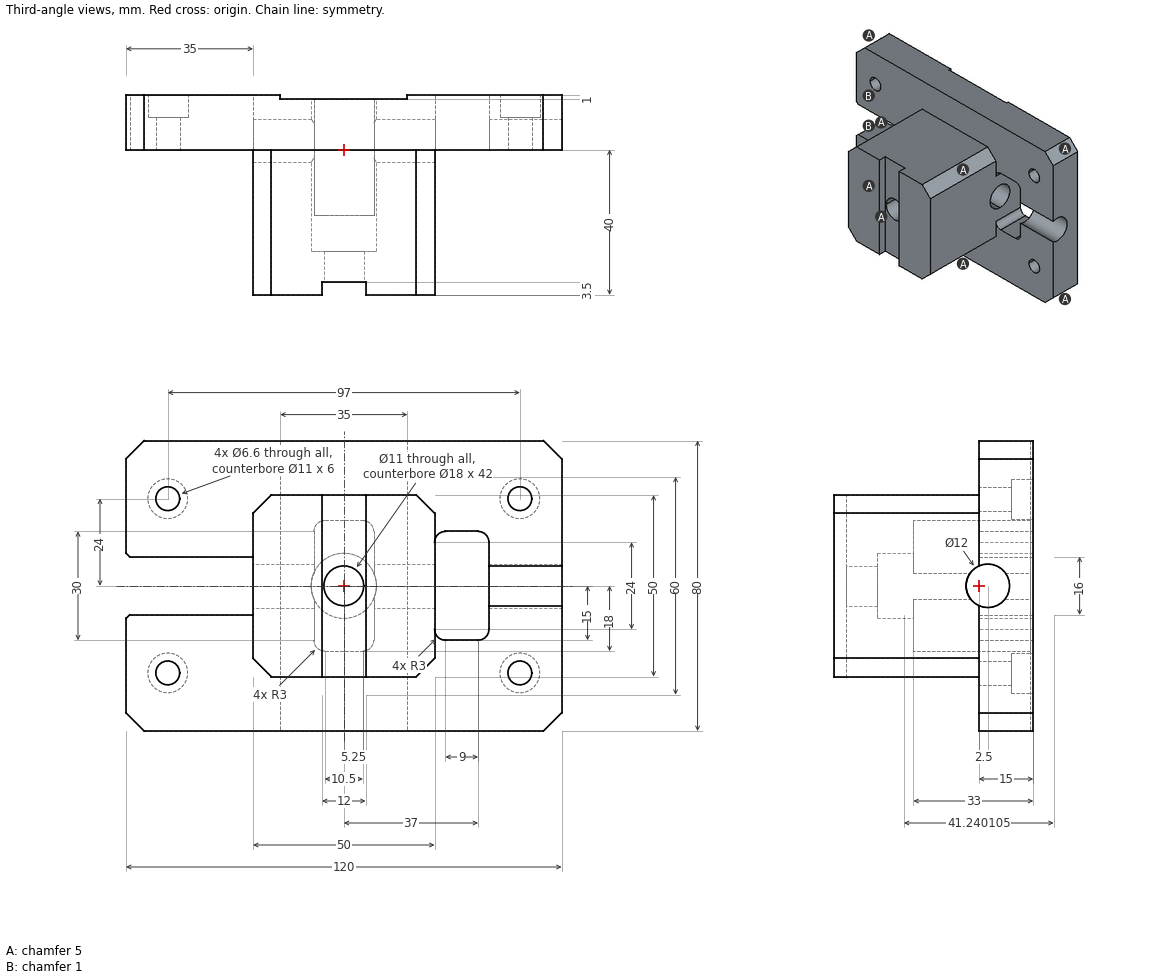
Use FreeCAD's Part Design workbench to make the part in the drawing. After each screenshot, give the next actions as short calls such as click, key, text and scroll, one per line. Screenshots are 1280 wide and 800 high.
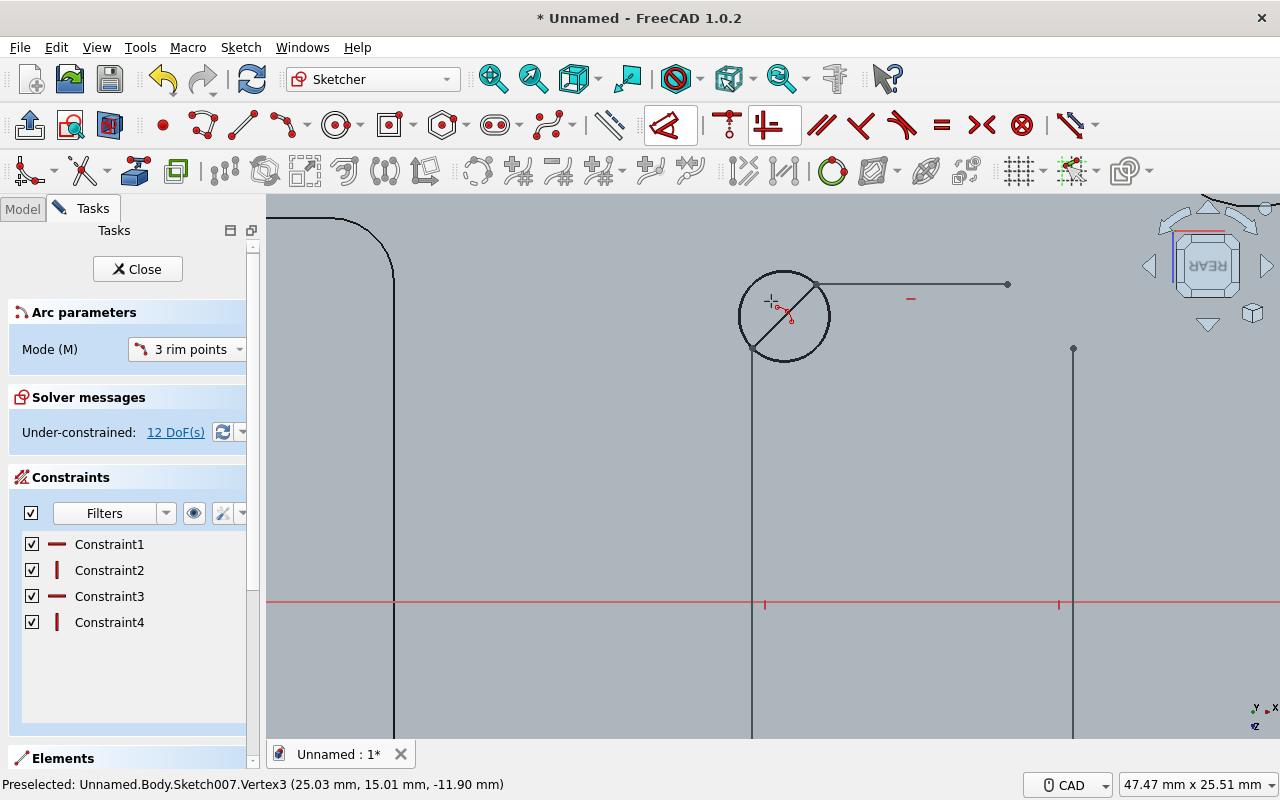
click(771, 301)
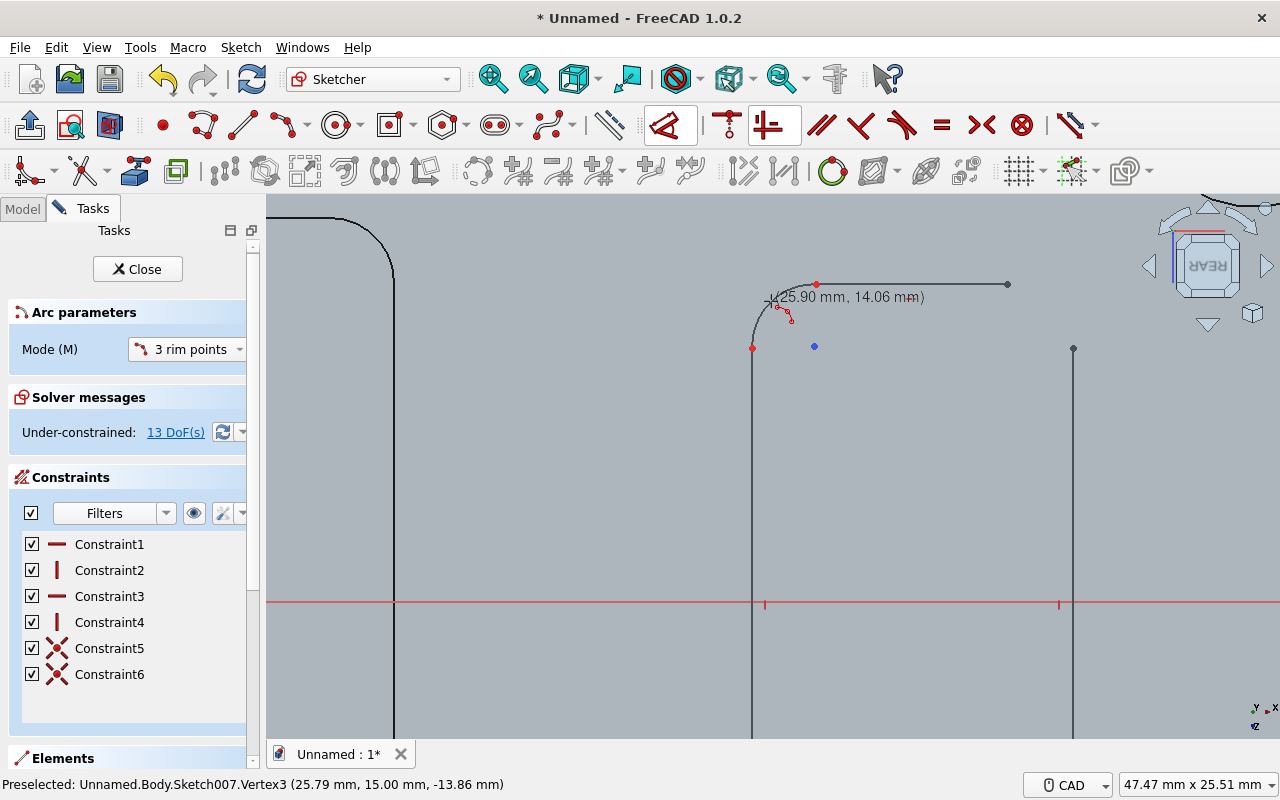
scroll(777, 301, down, 3)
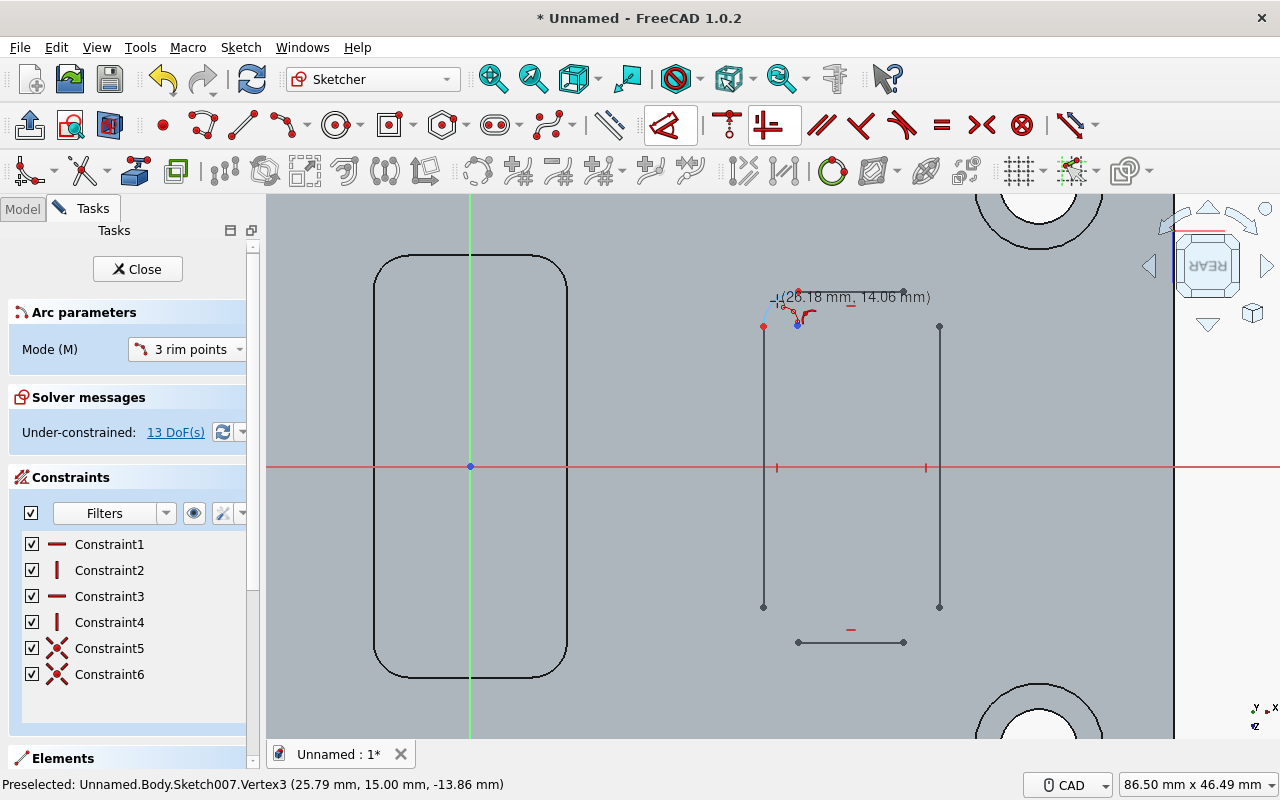
click(764, 608)
click(799, 643)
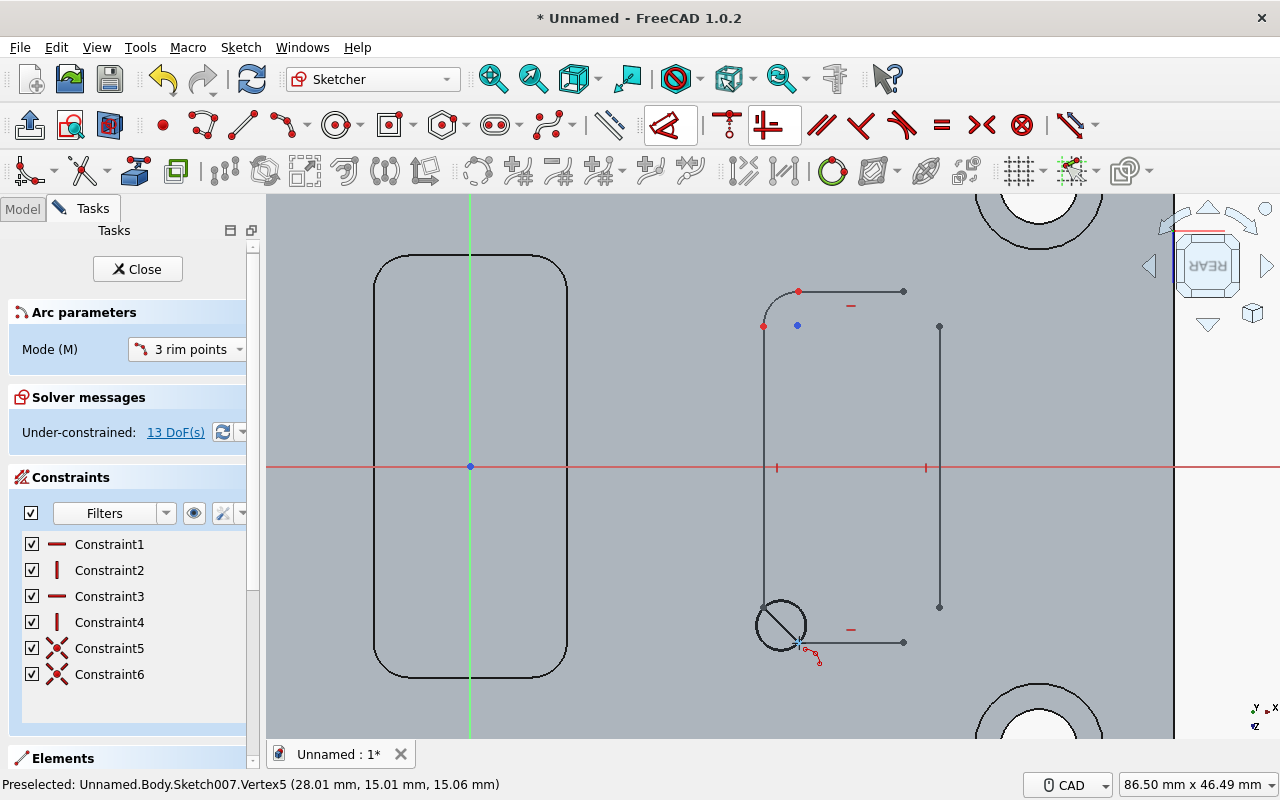
scroll(774, 632, up, 3)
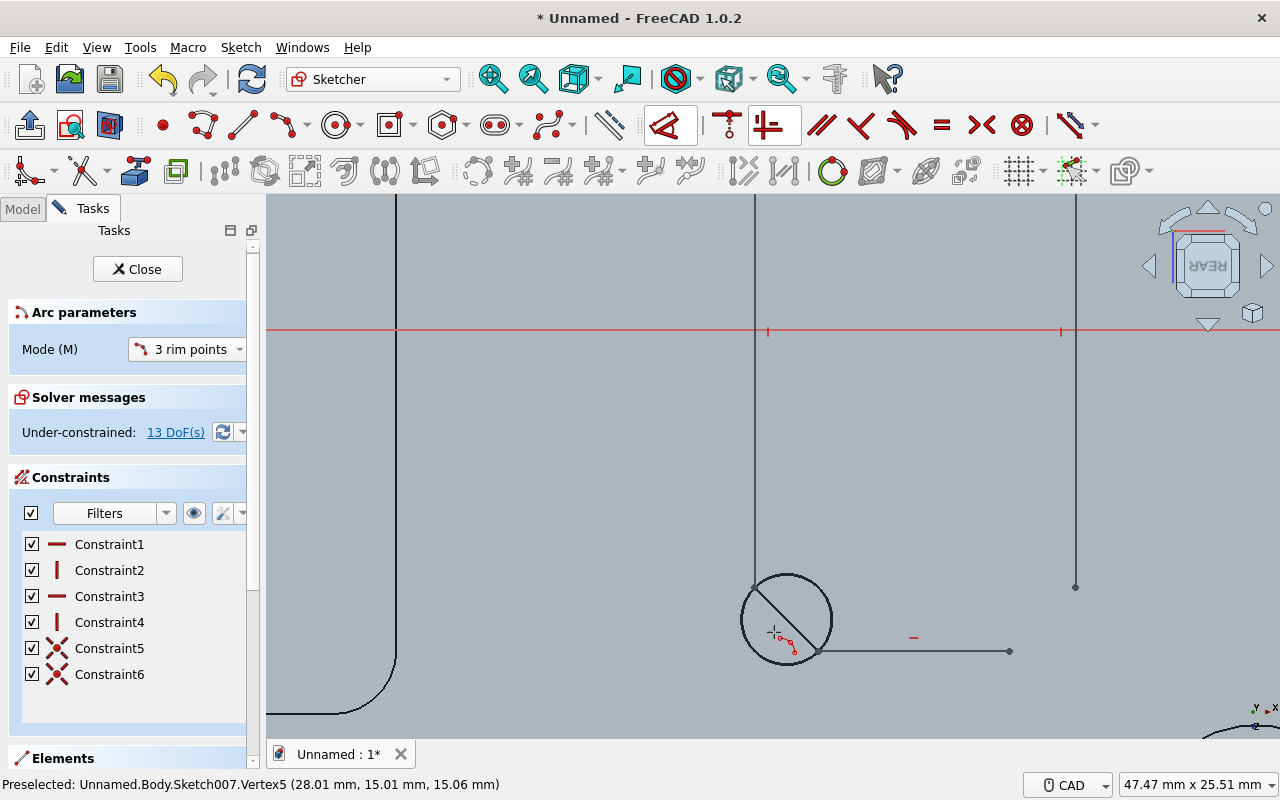
click(773, 631)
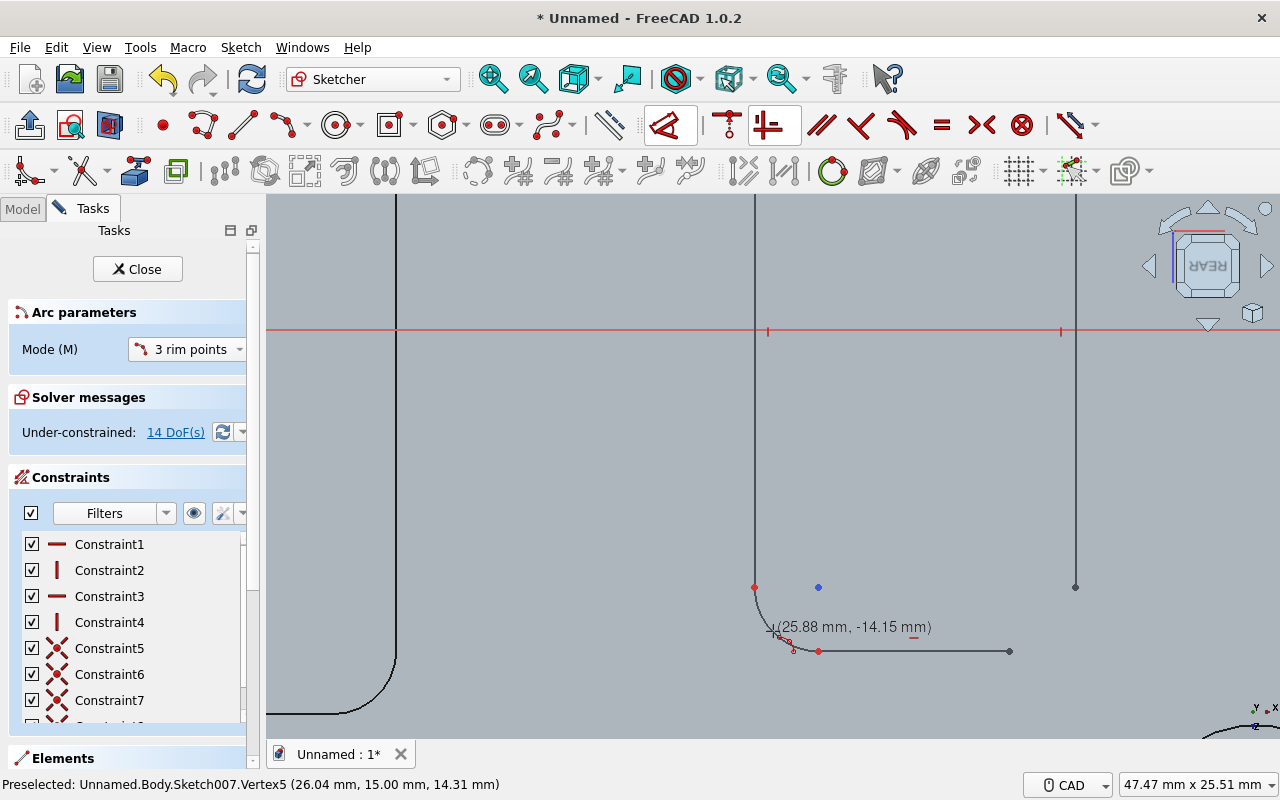
click(1010, 651)
click(1076, 588)
click(1056, 631)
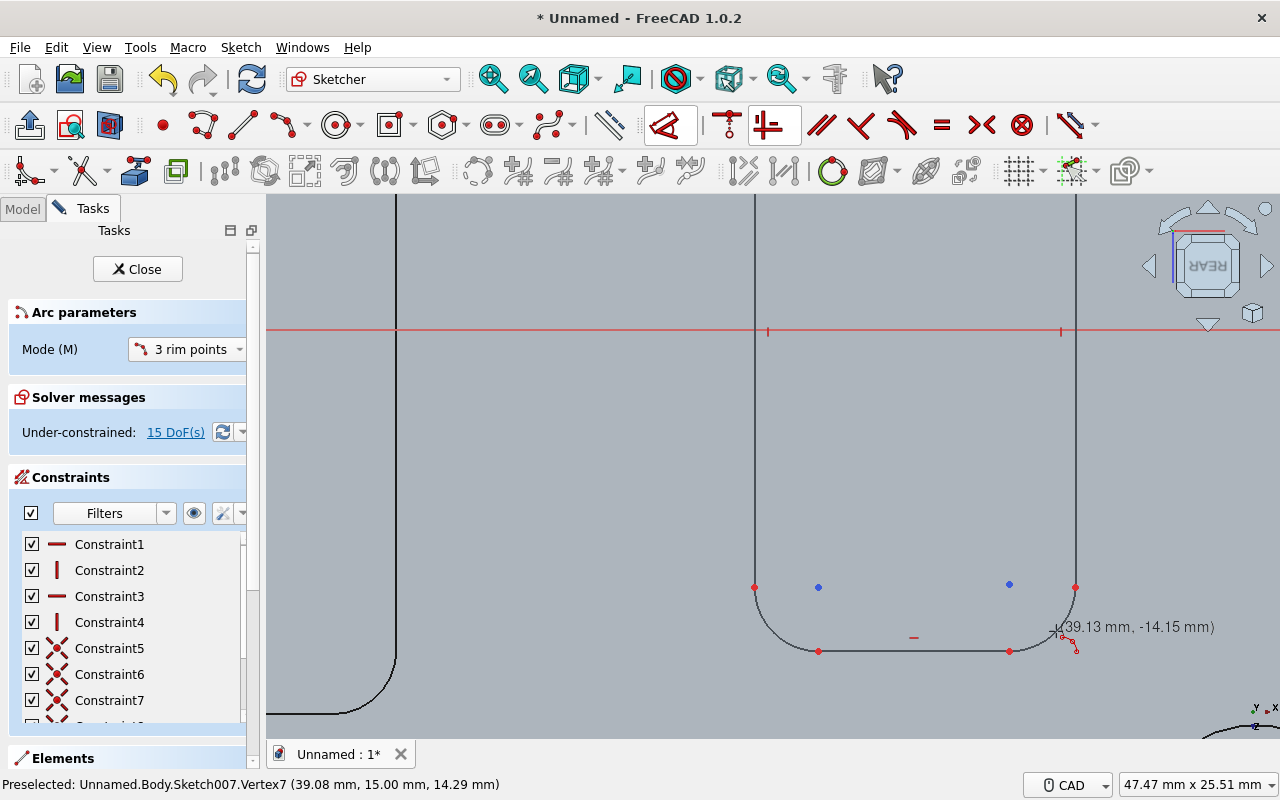
scroll(774, 633, down, 3)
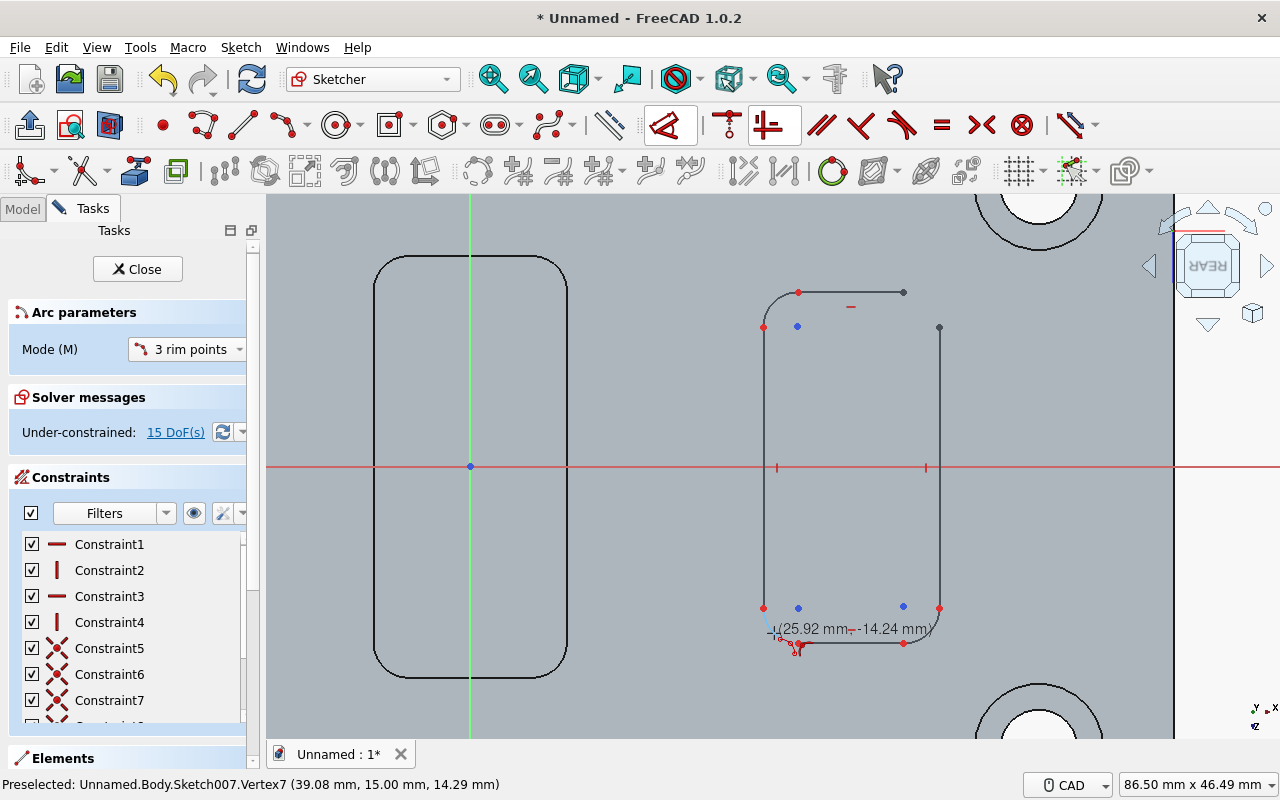
click(940, 327)
click(904, 292)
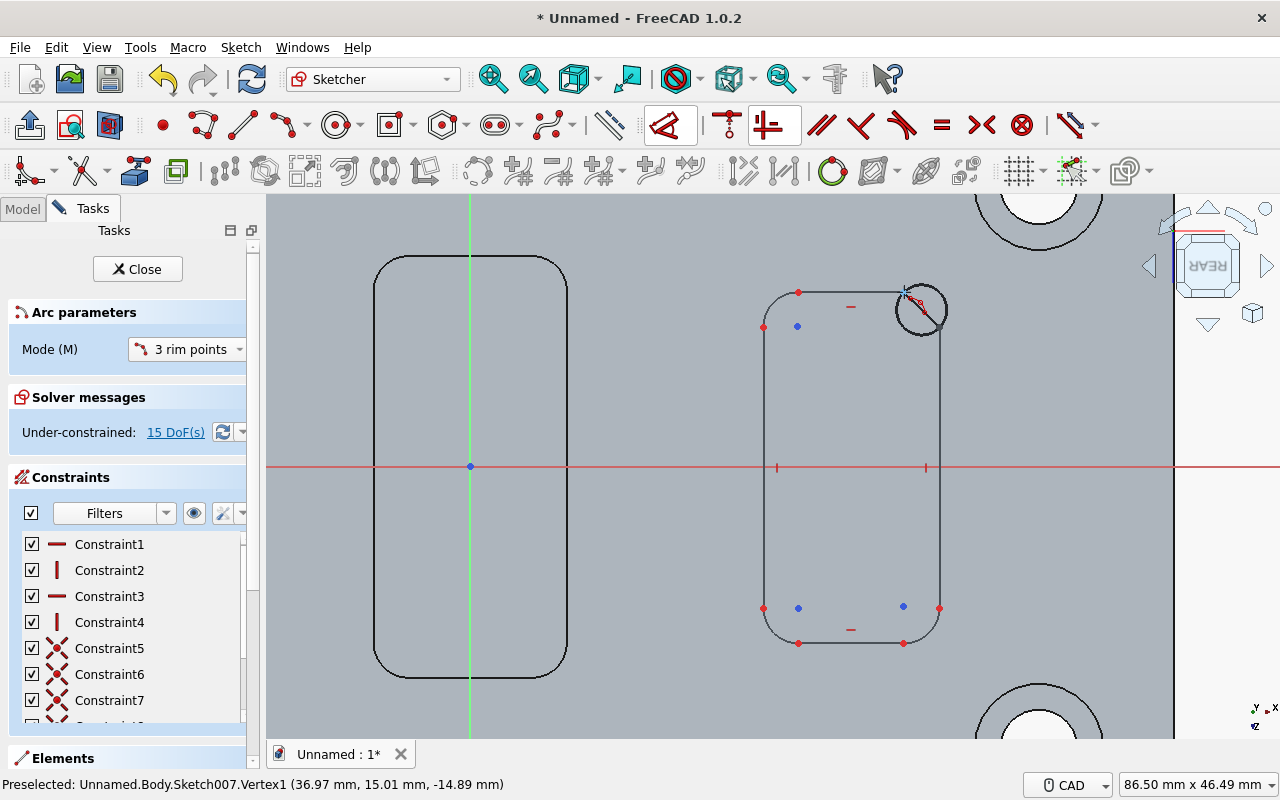
scroll(929, 301, up, 3)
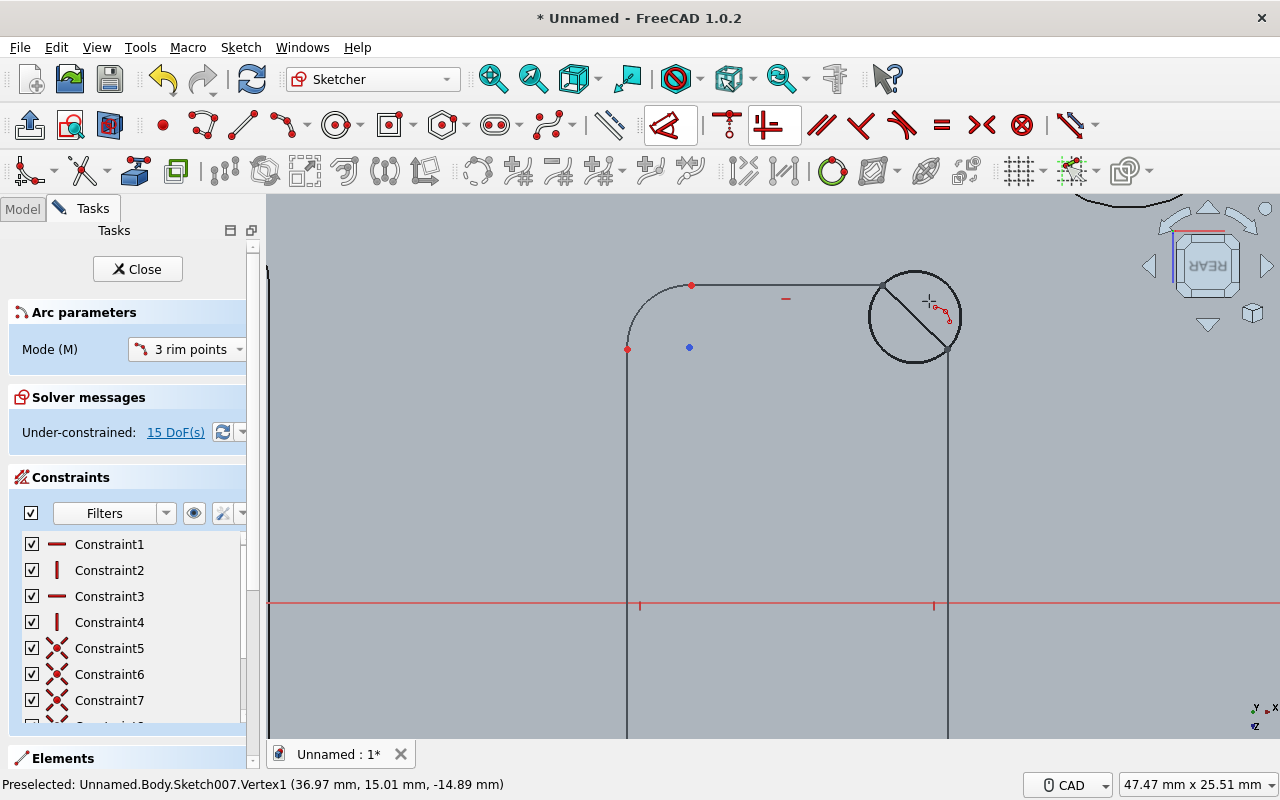
click(928, 302)
key(Escape)